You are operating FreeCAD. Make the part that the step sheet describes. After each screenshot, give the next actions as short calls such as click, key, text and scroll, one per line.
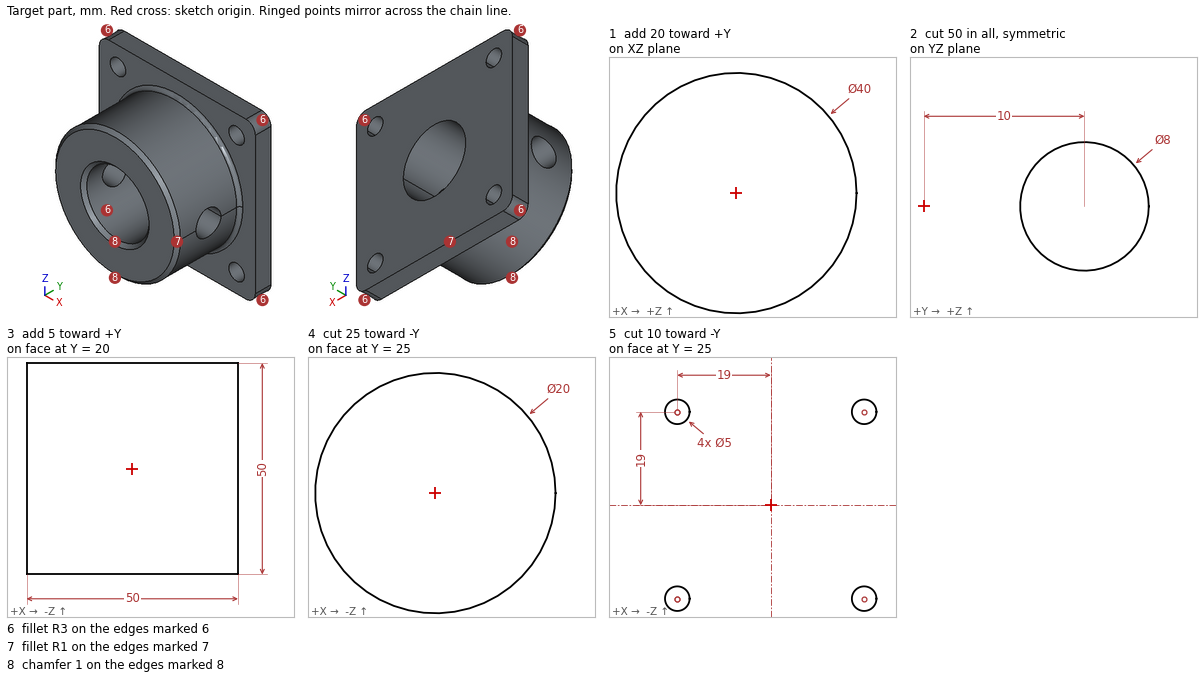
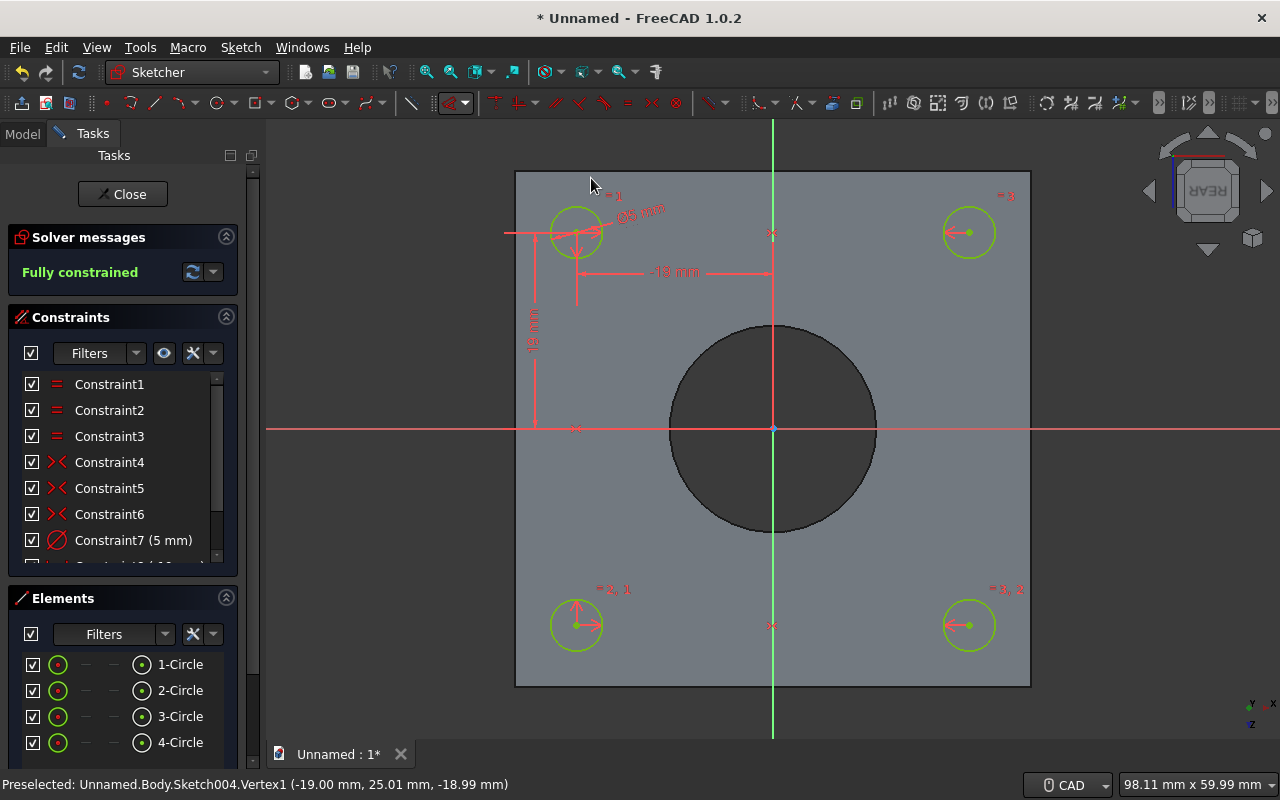
click(123, 194)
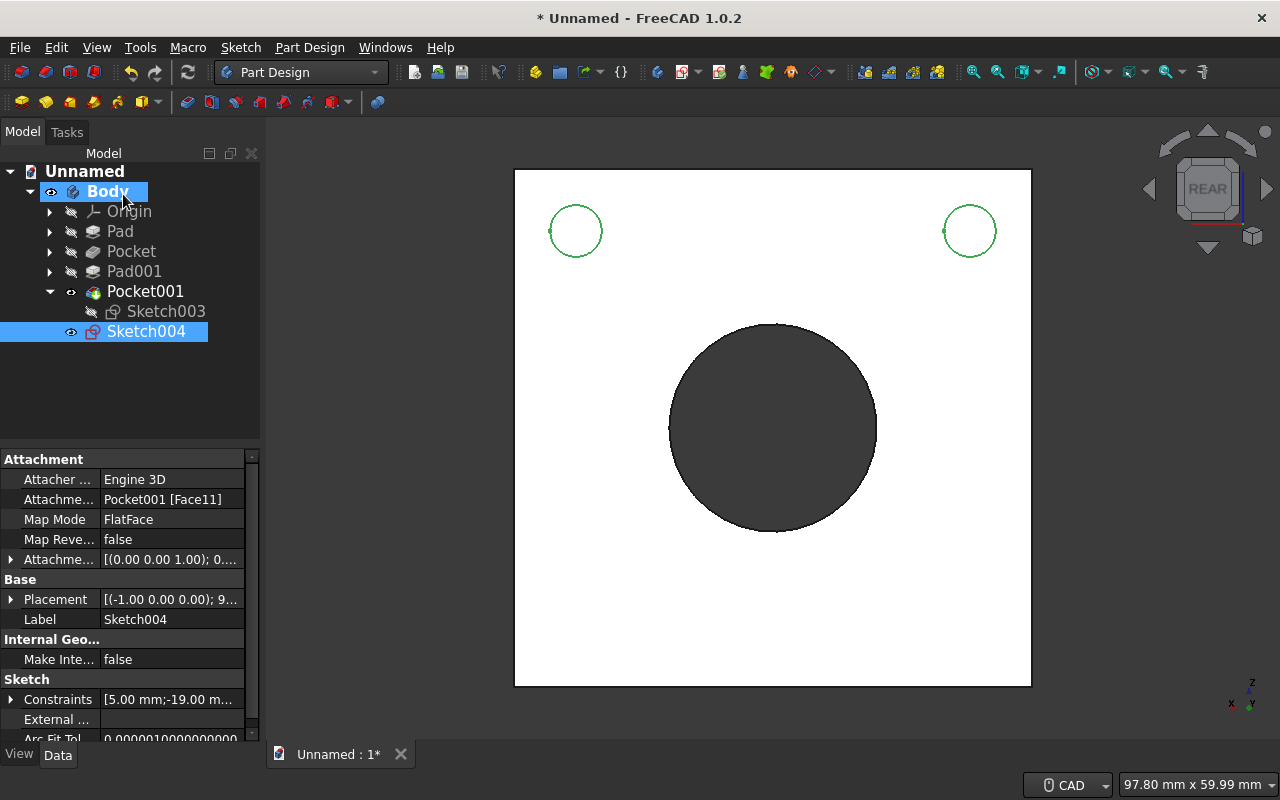
click(188, 102)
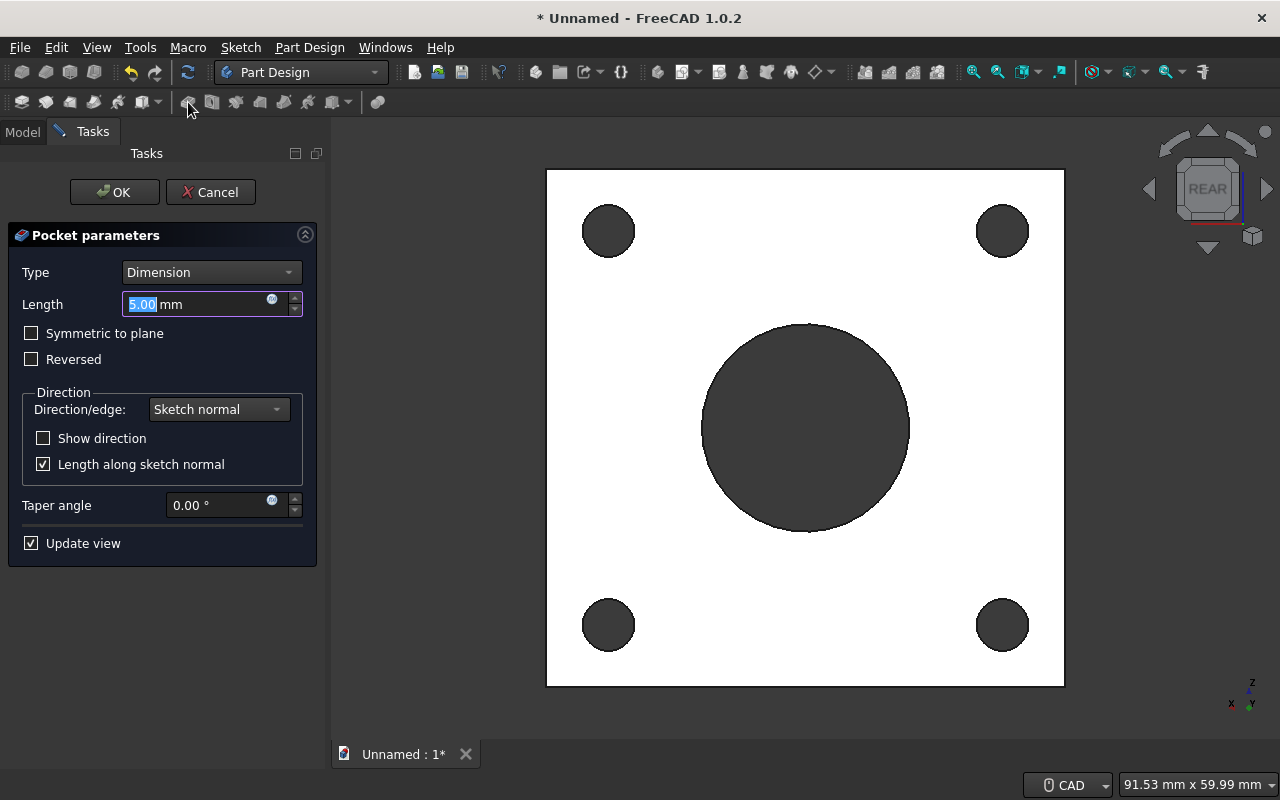
text(10)
key(Tab)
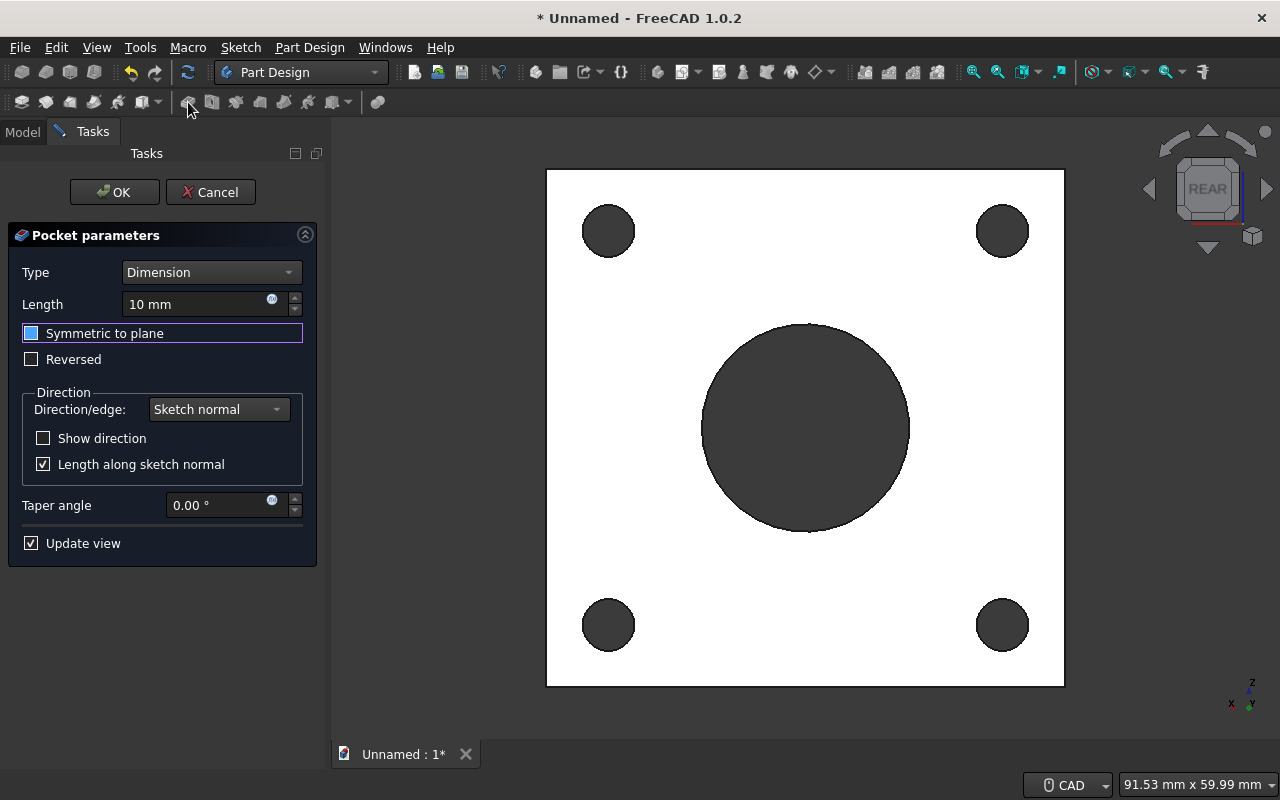
click(115, 192)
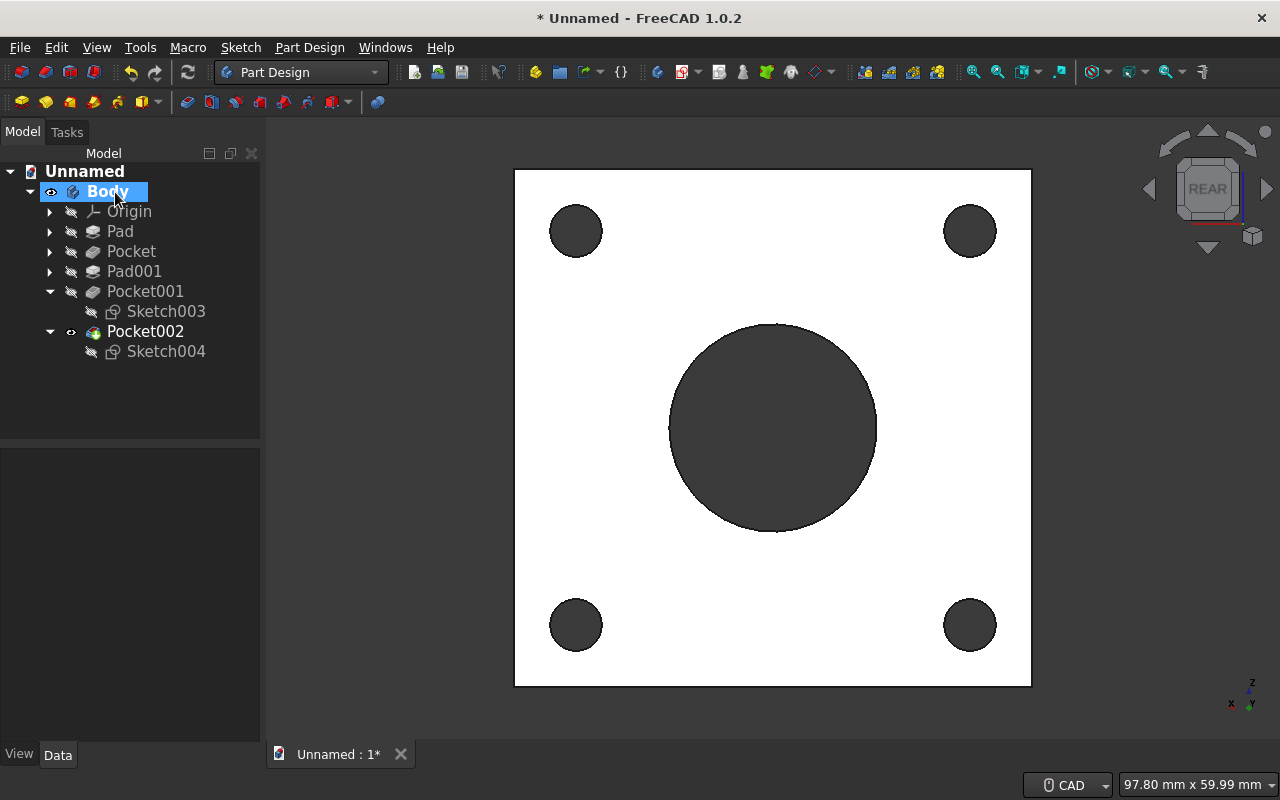
key(0)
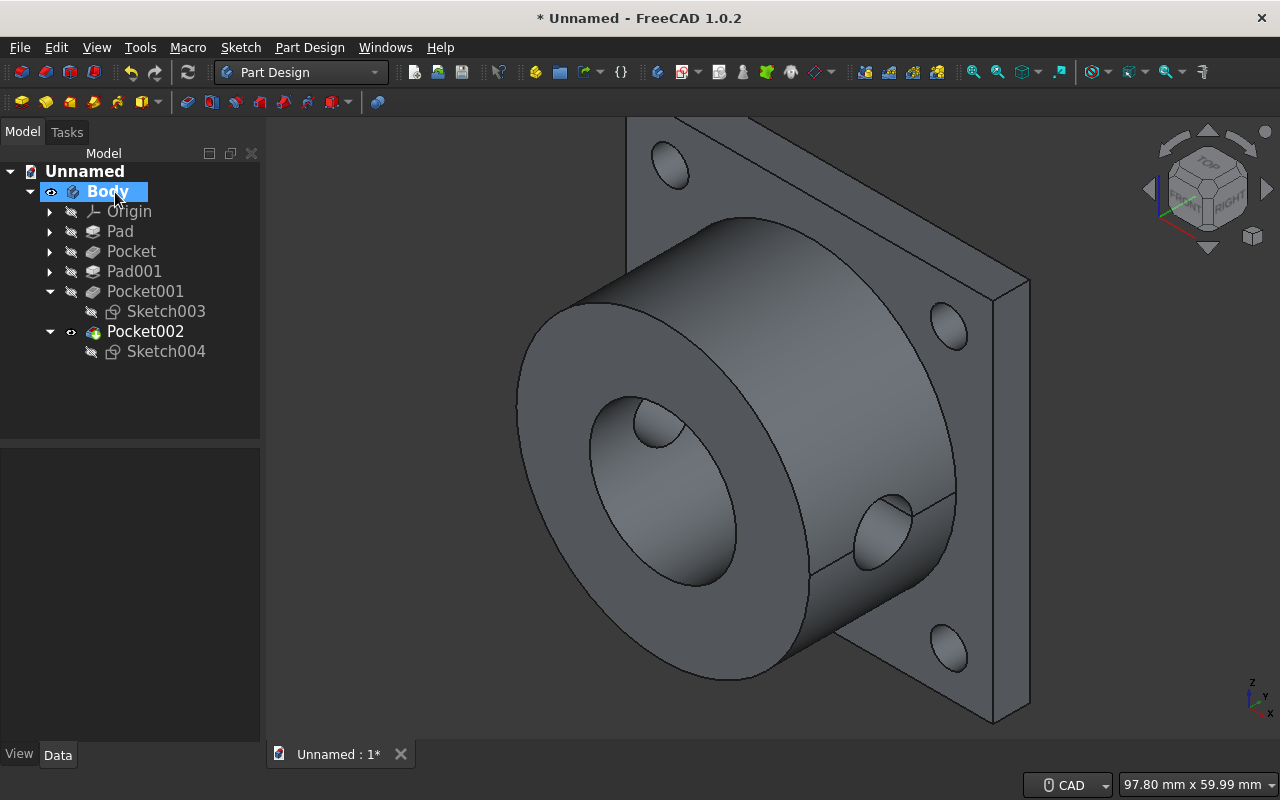
key(v)
key(f)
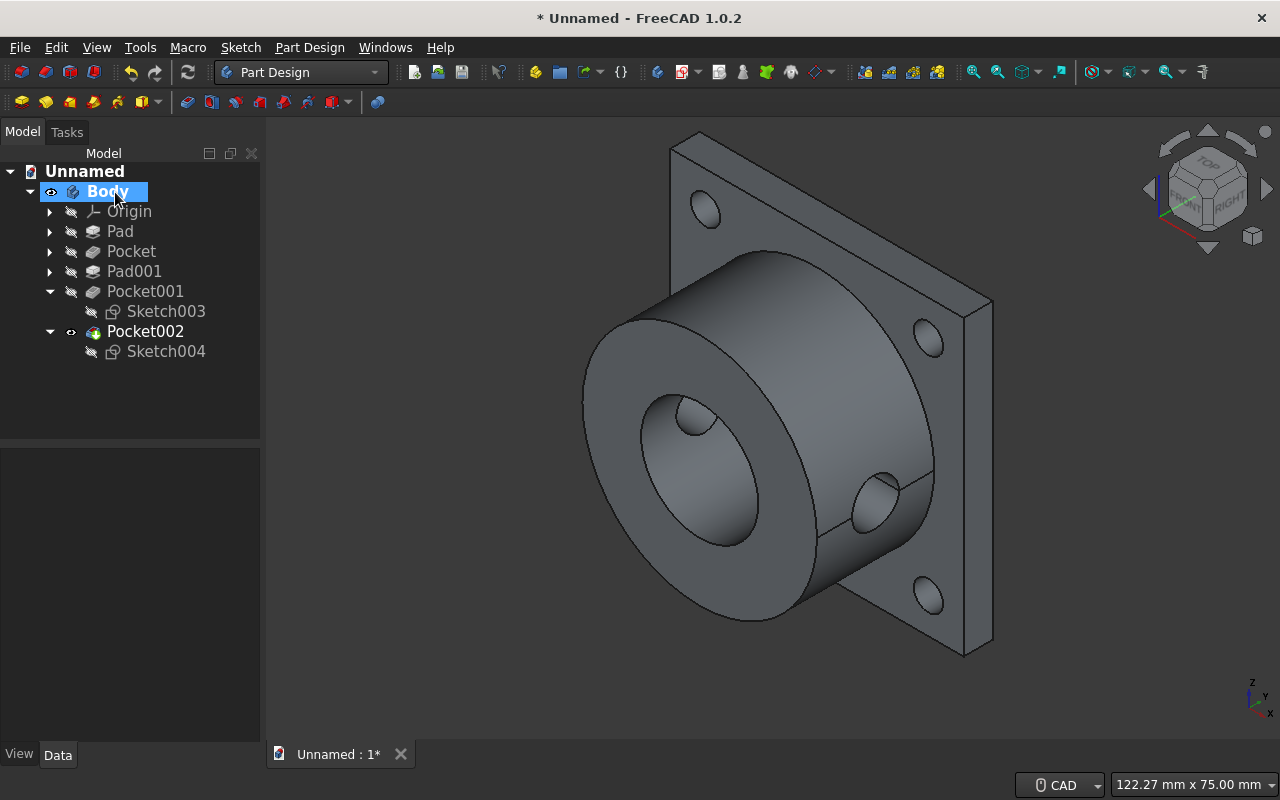
click(978, 308)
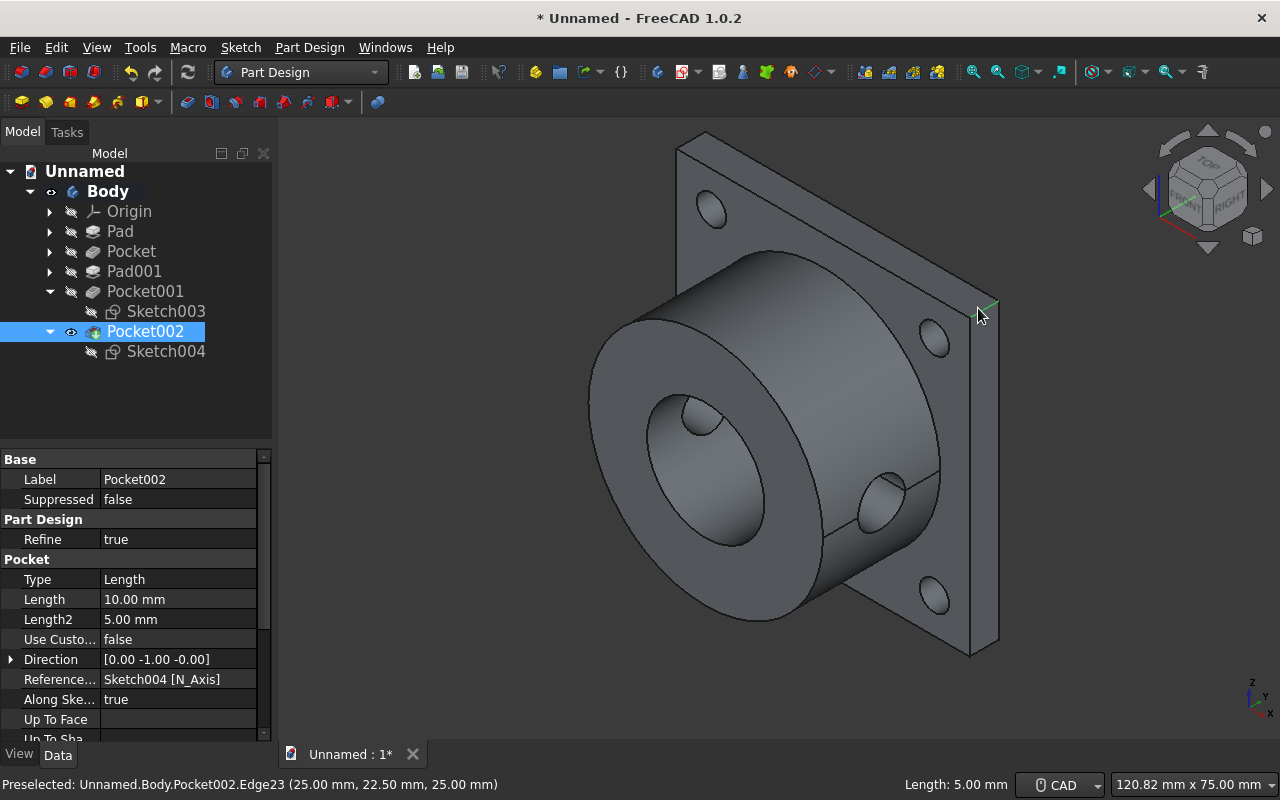
key(2)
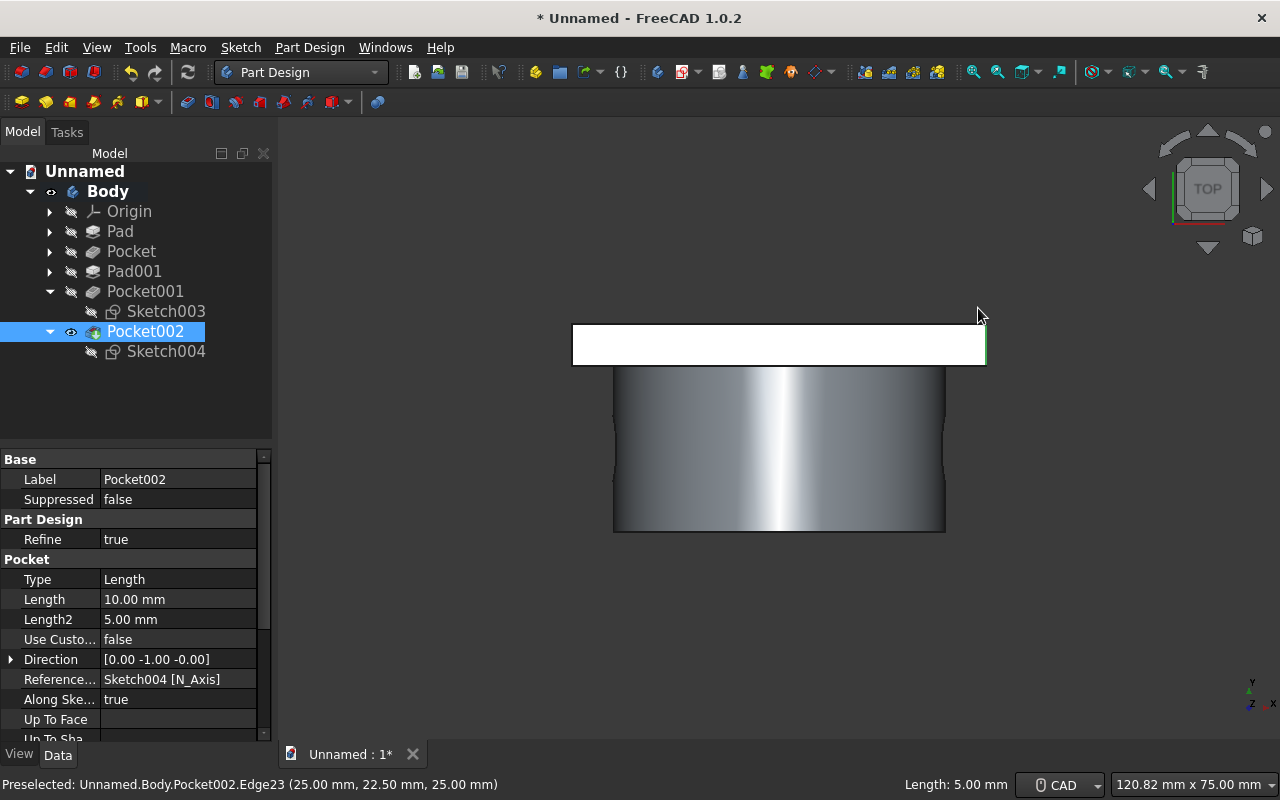
key(v)
key(f)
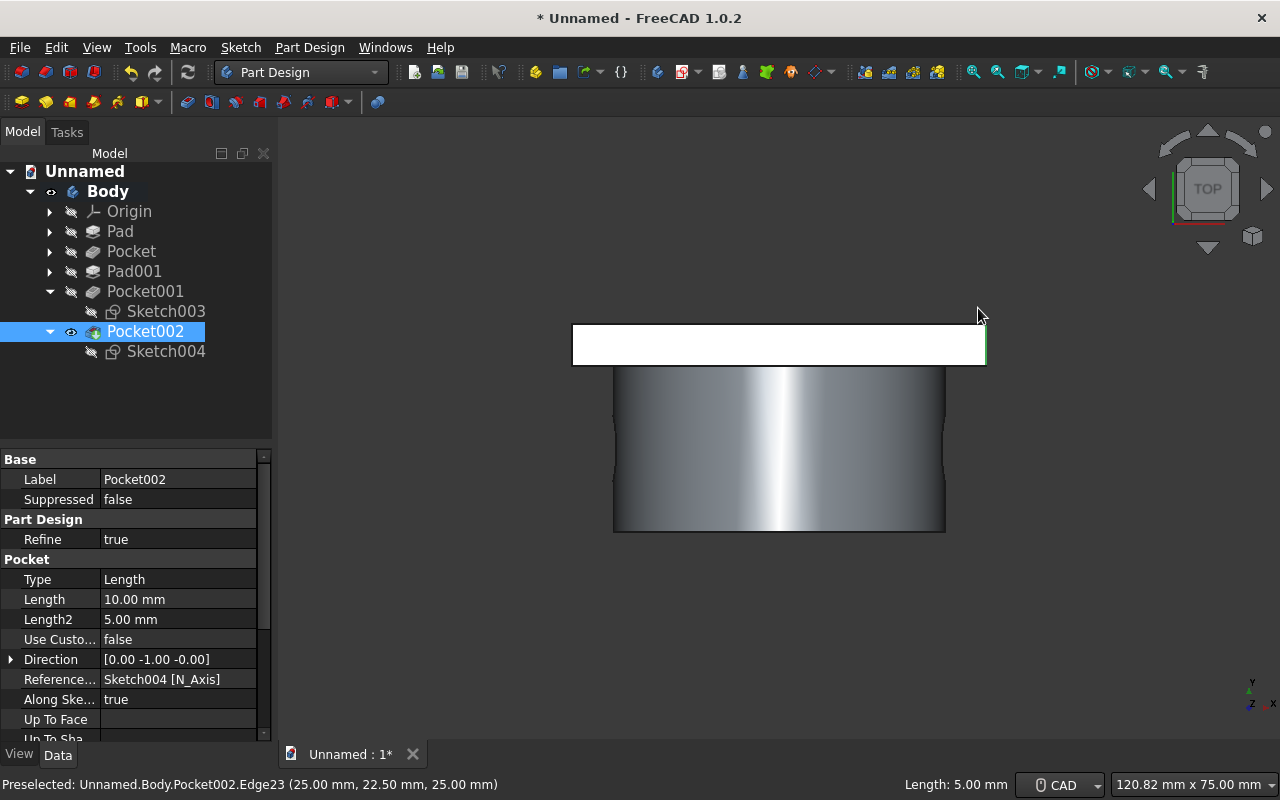
click(572, 344, ctrl)